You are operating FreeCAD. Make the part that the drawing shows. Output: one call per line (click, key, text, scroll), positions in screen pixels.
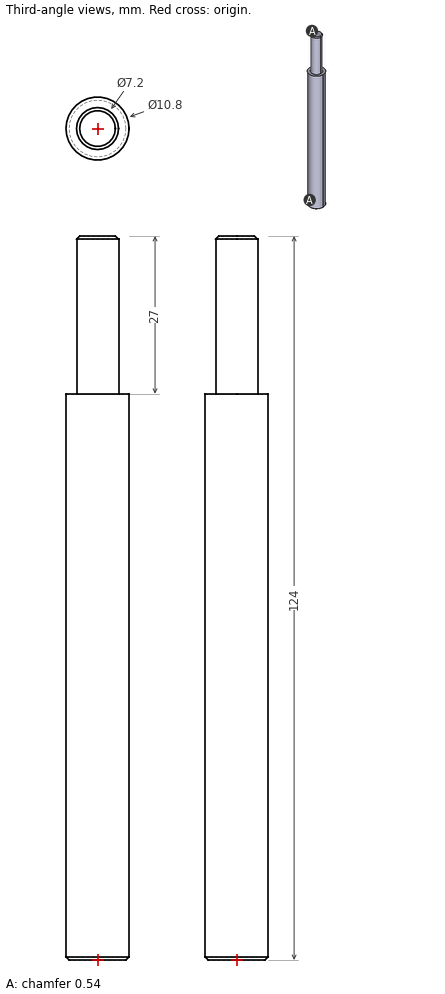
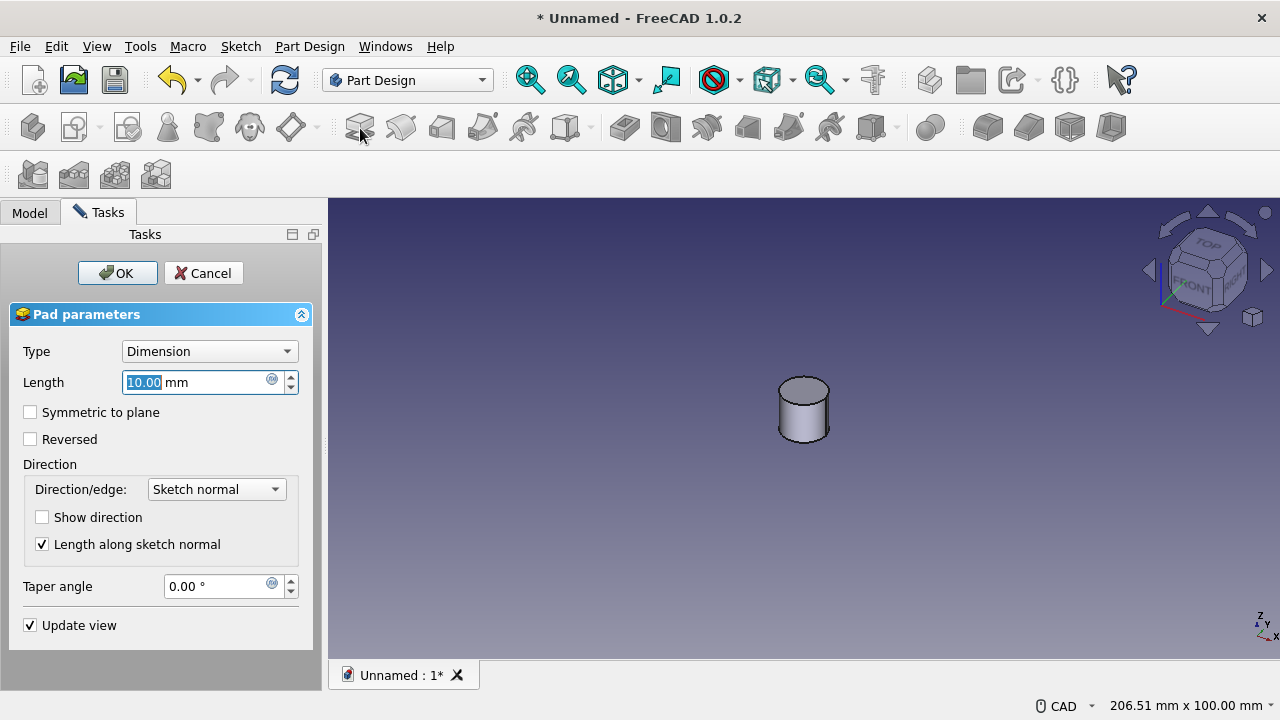
text(124)
key(Tab)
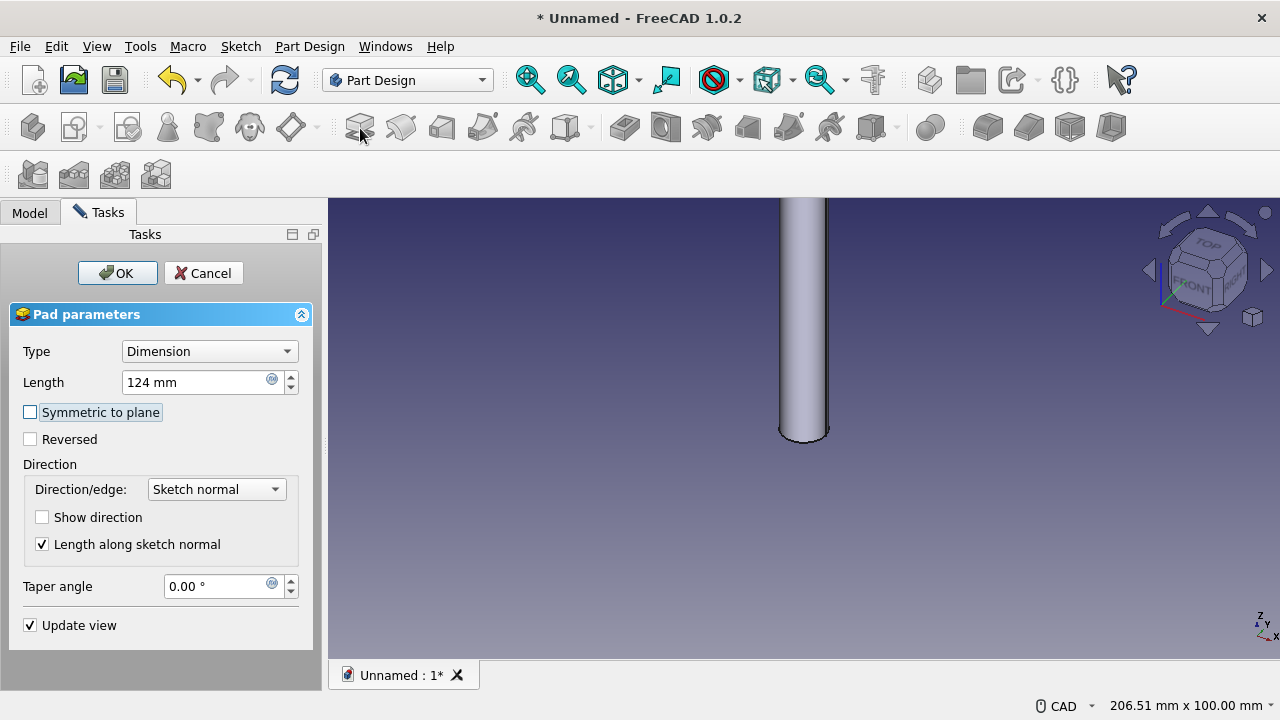
click(118, 273)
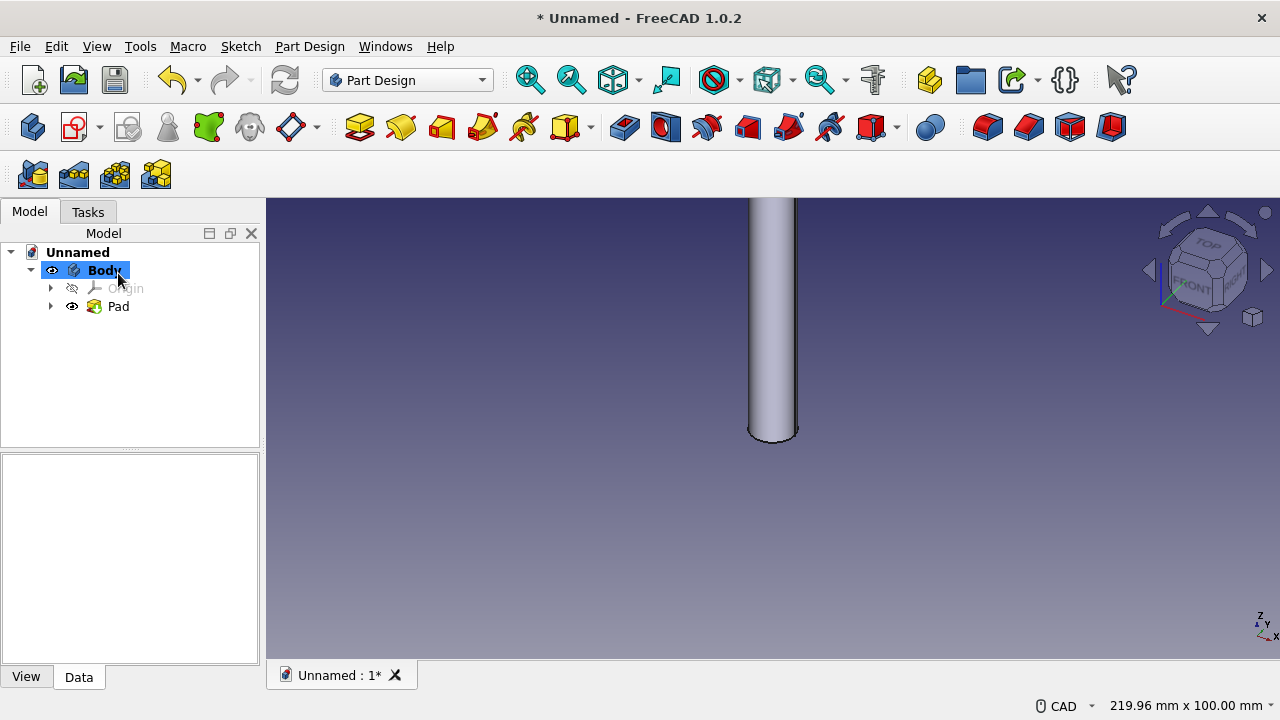
click(531, 80)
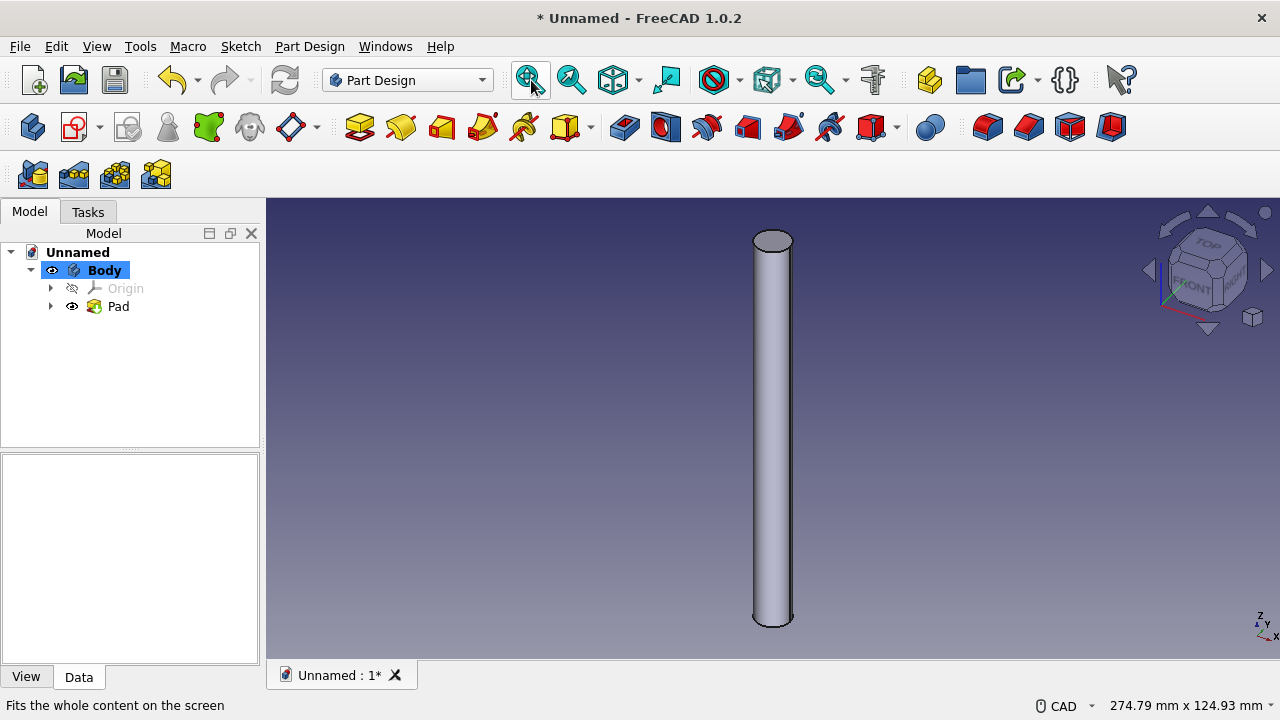
click(51, 288)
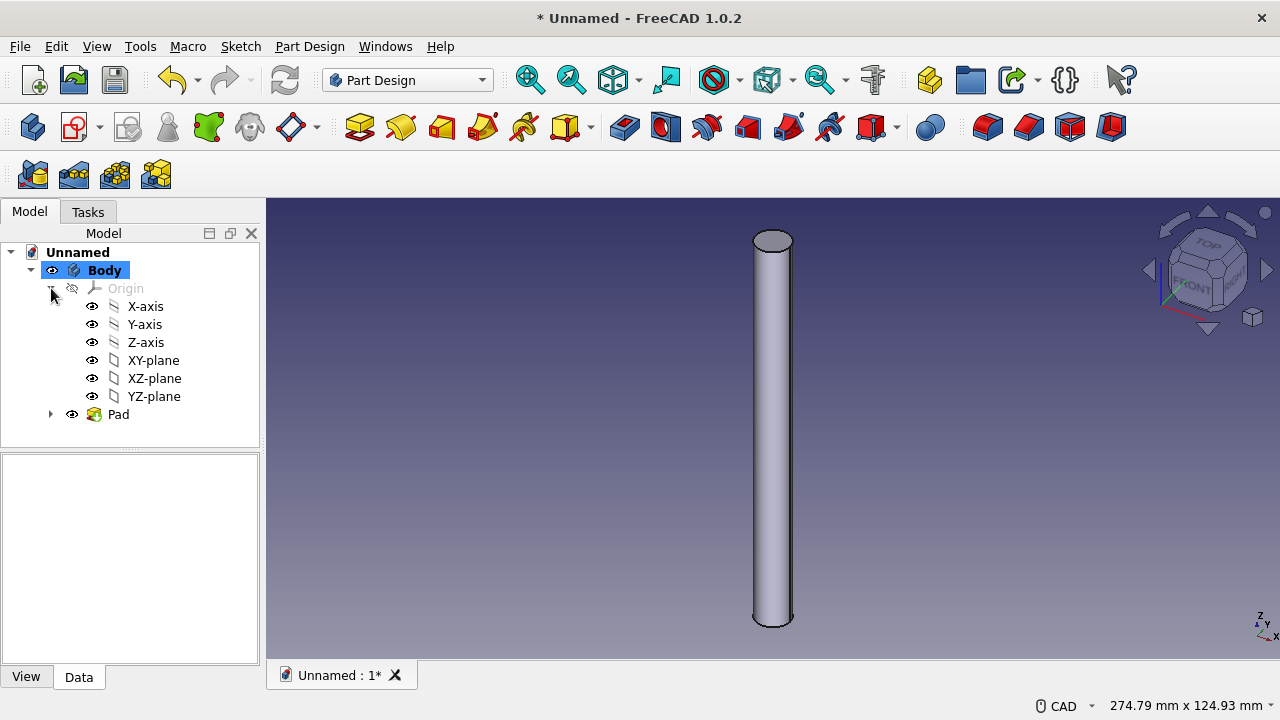
click(137, 360)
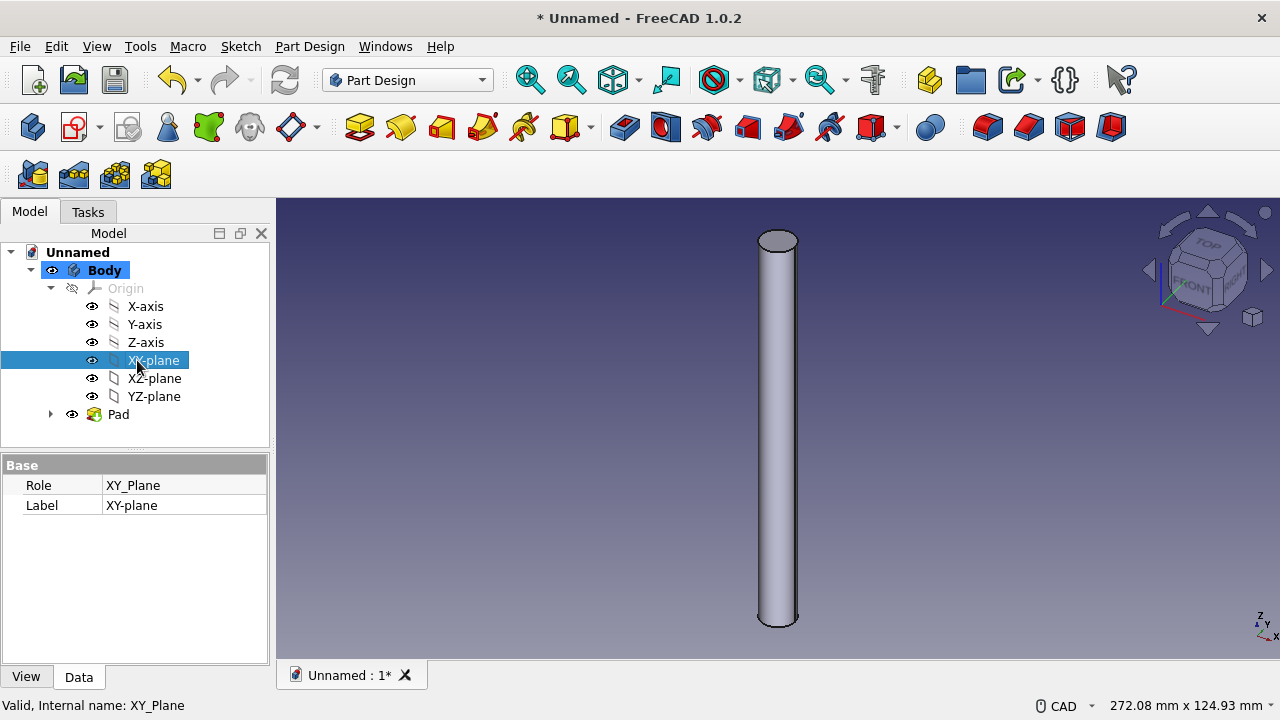
click(290, 128)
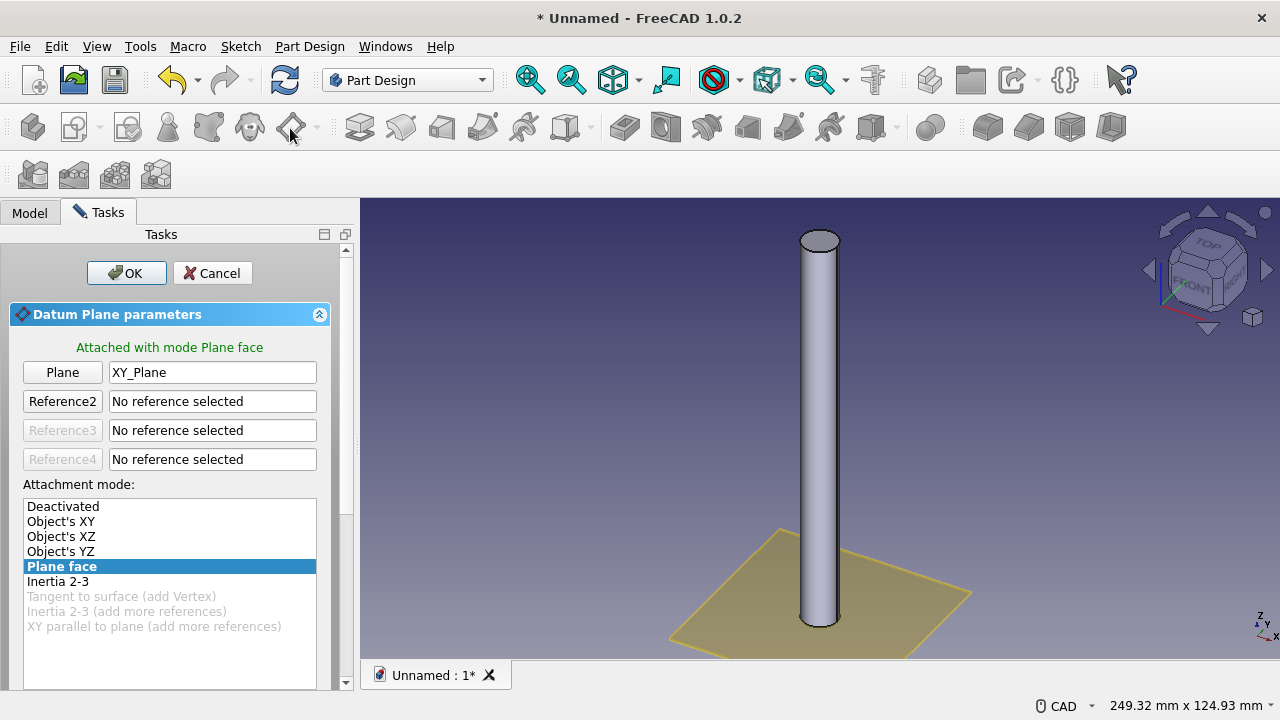
scroll(346, 467, down, 4)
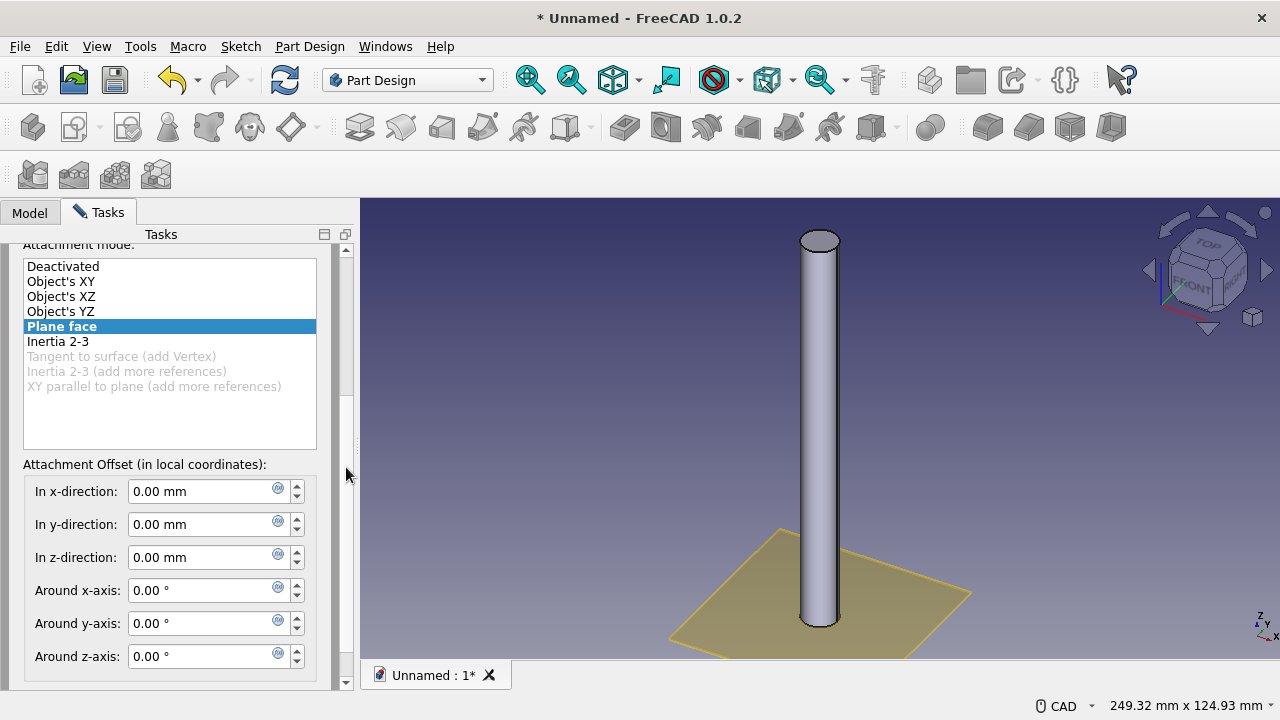
triple_click(210, 558)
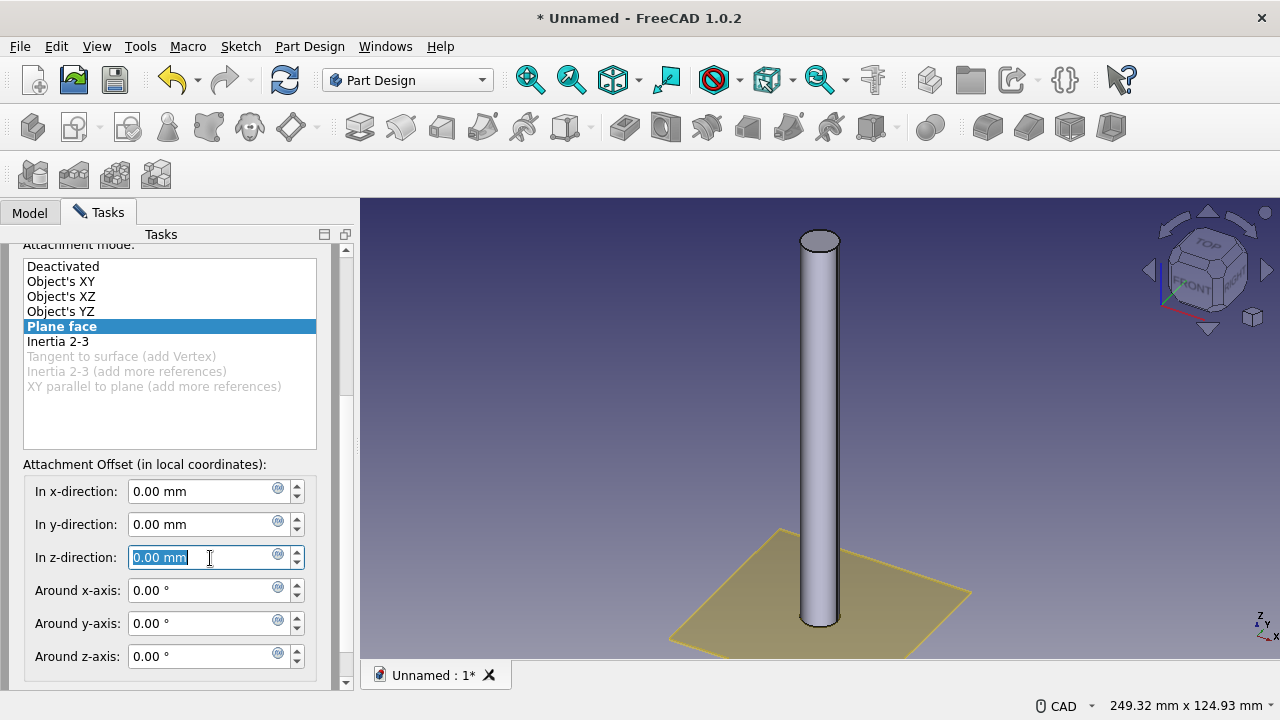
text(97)
key(Tab)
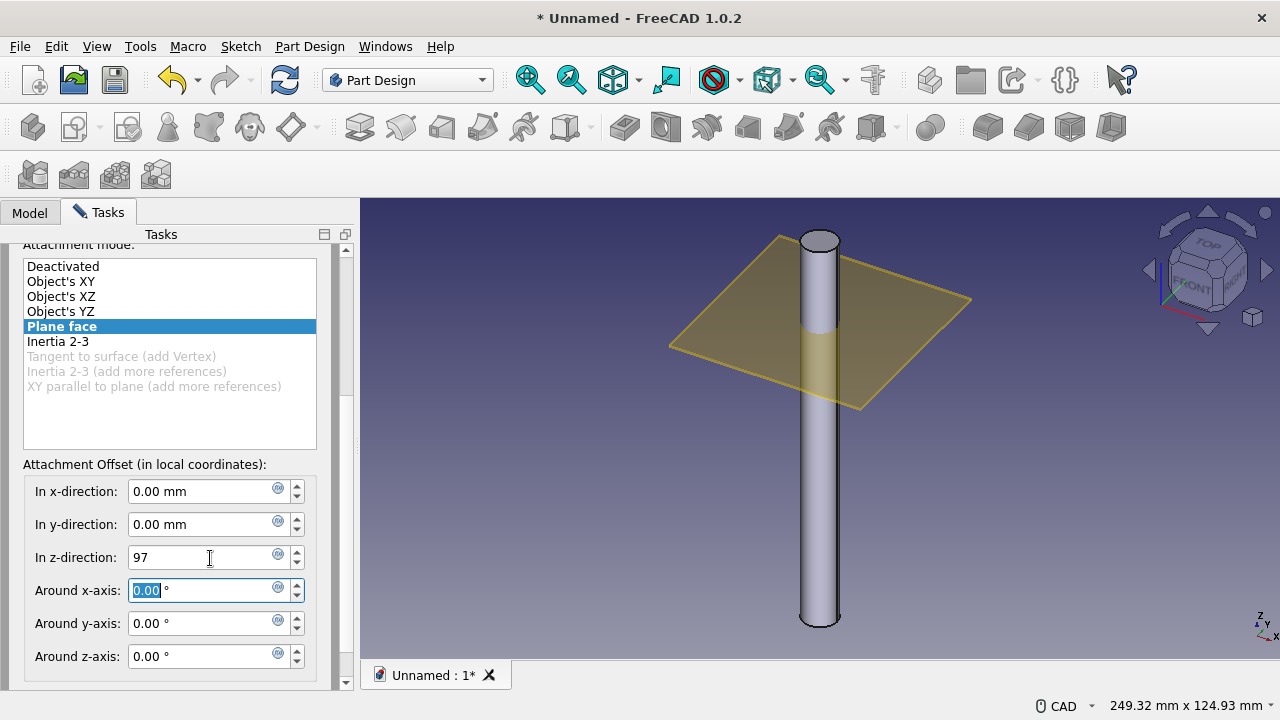
scroll(346, 467, up, 5)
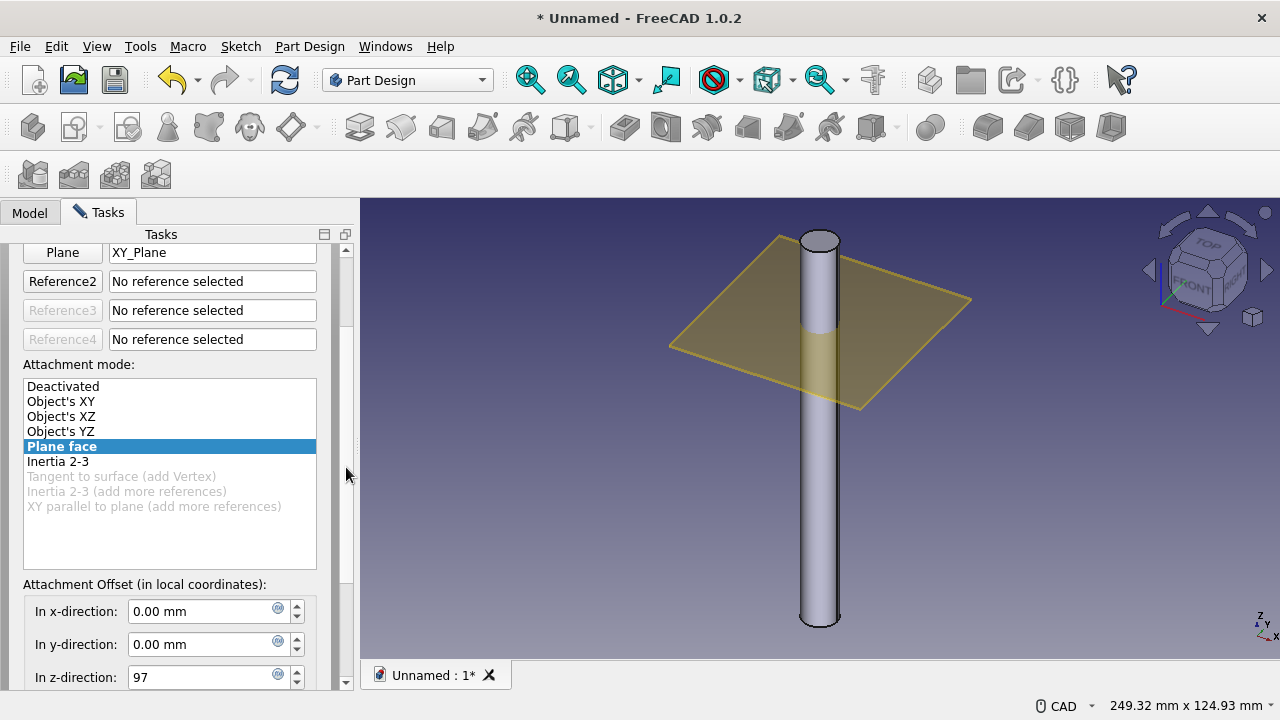
click(127, 273)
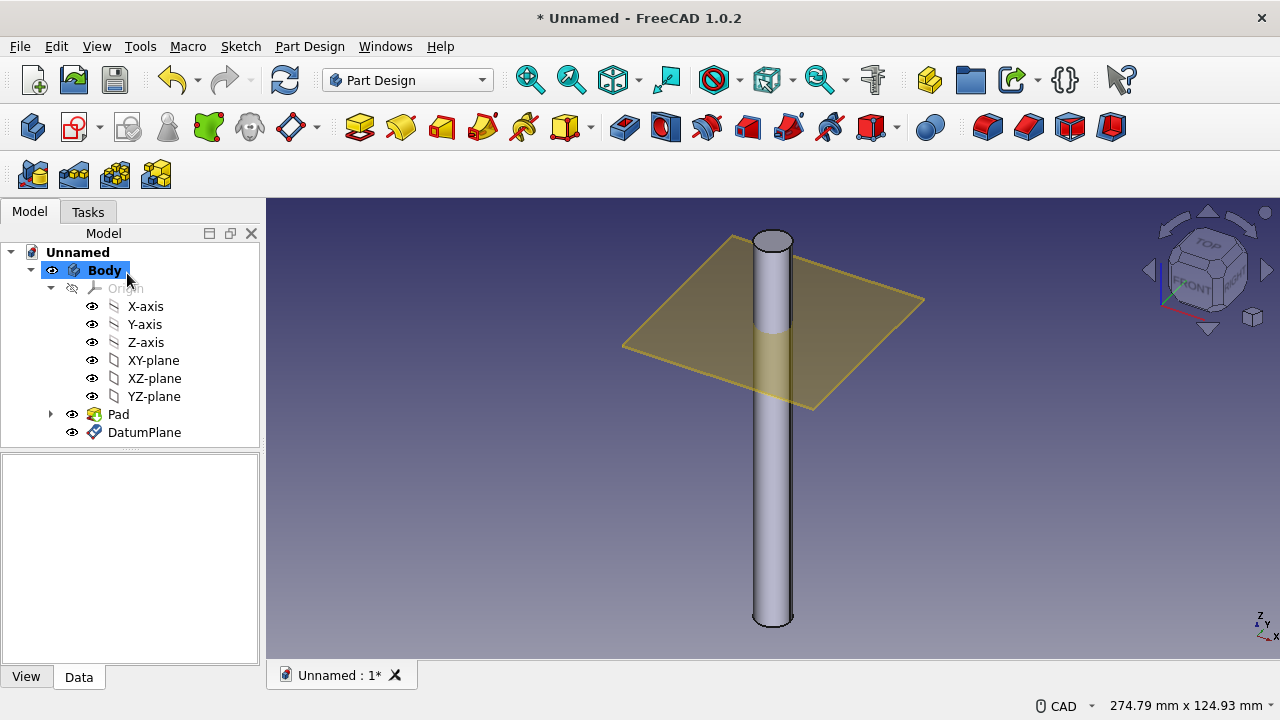
click(117, 432)